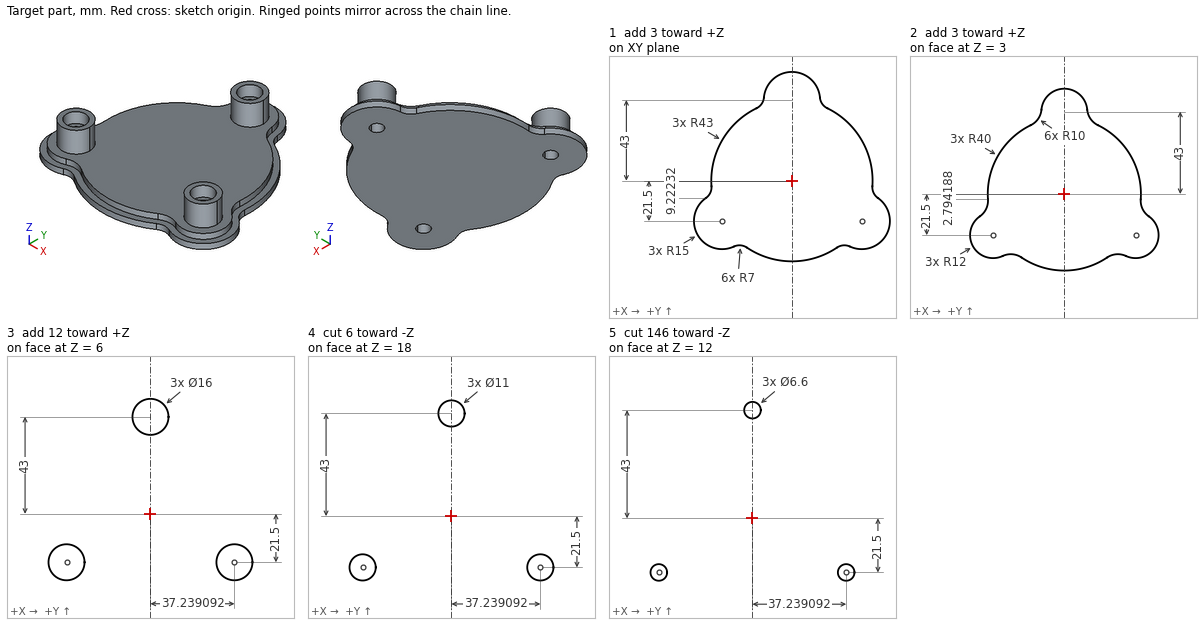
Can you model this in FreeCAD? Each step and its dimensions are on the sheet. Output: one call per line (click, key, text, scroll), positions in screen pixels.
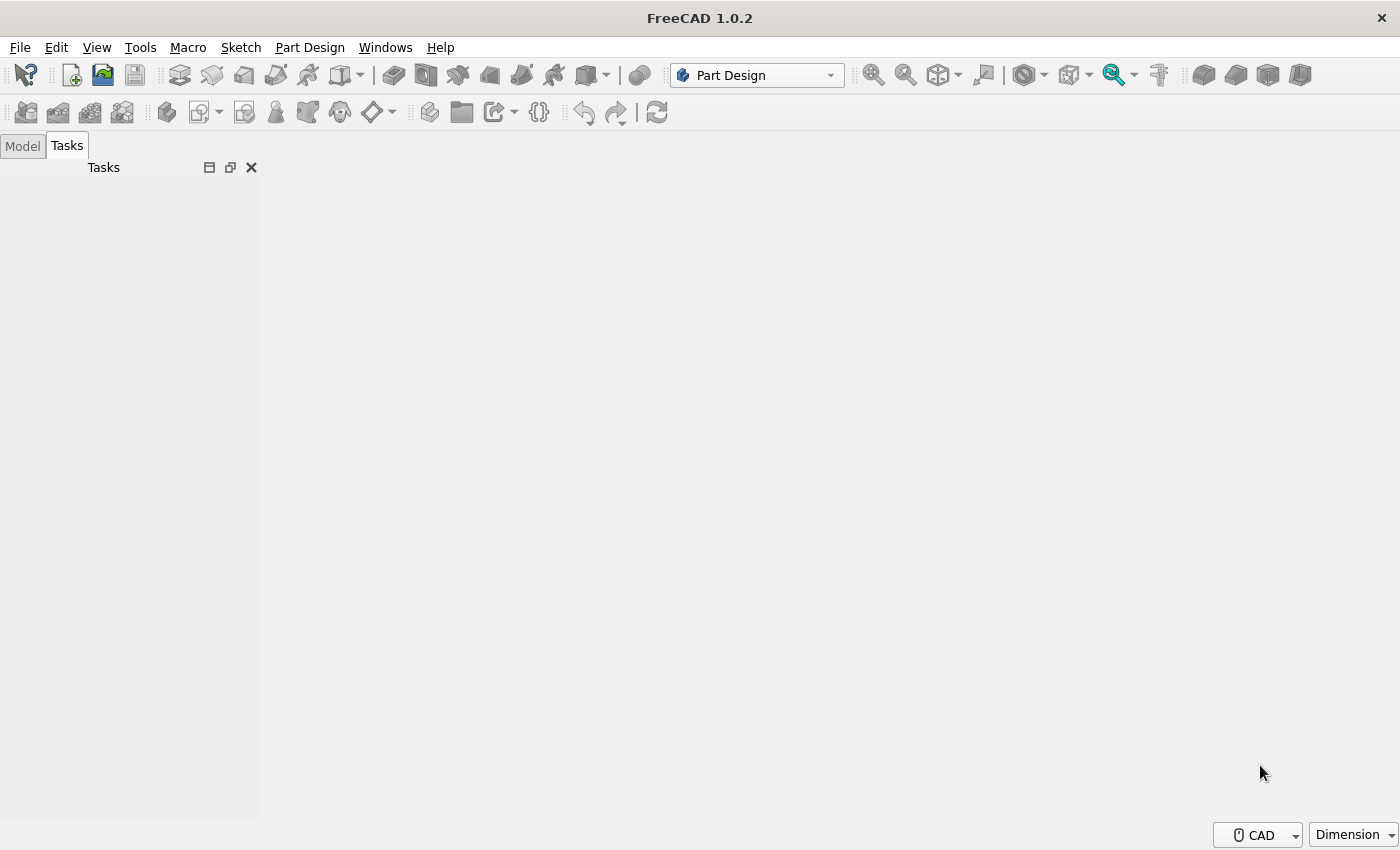
click(72, 76)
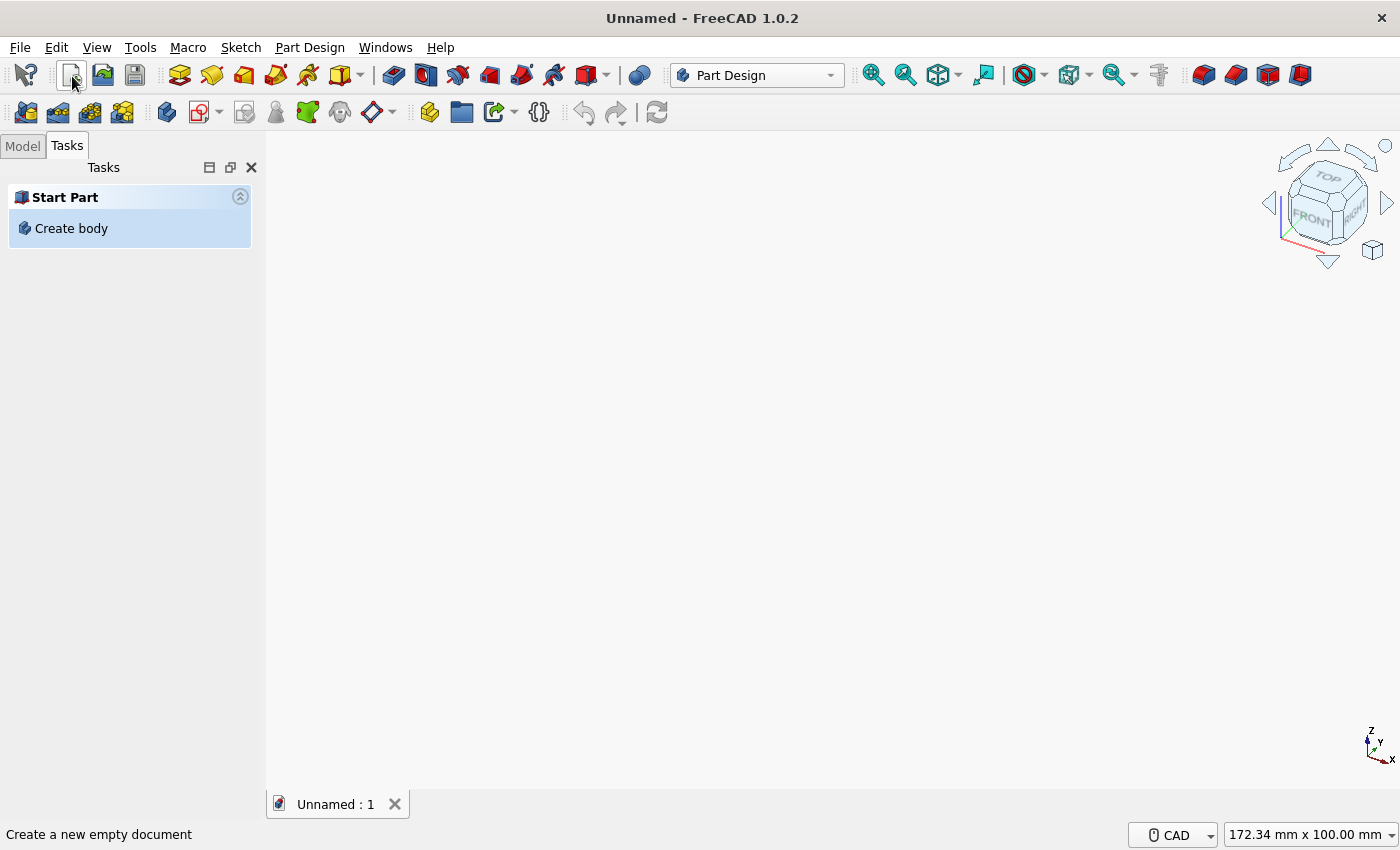
click(200, 112)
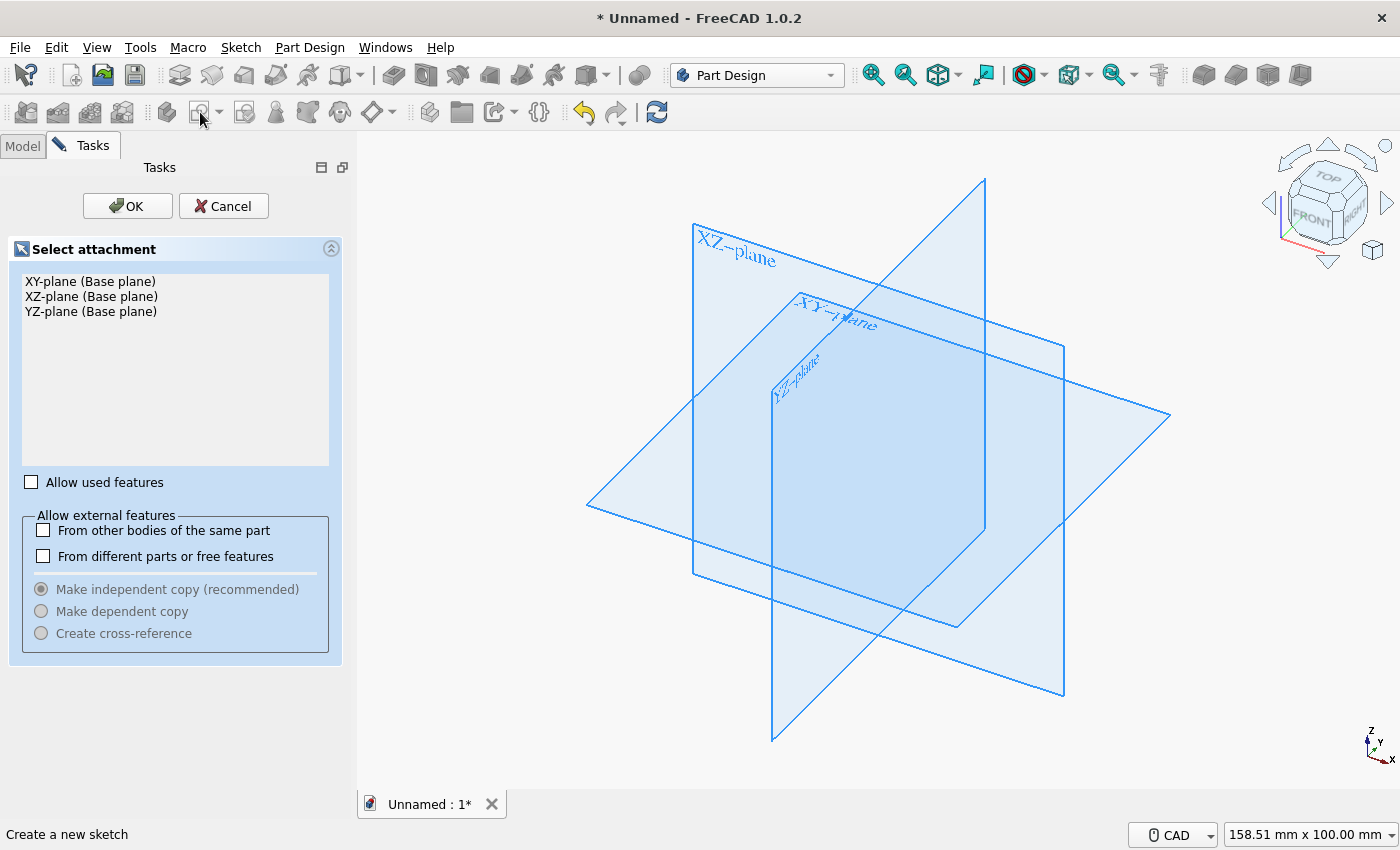
click(82, 282)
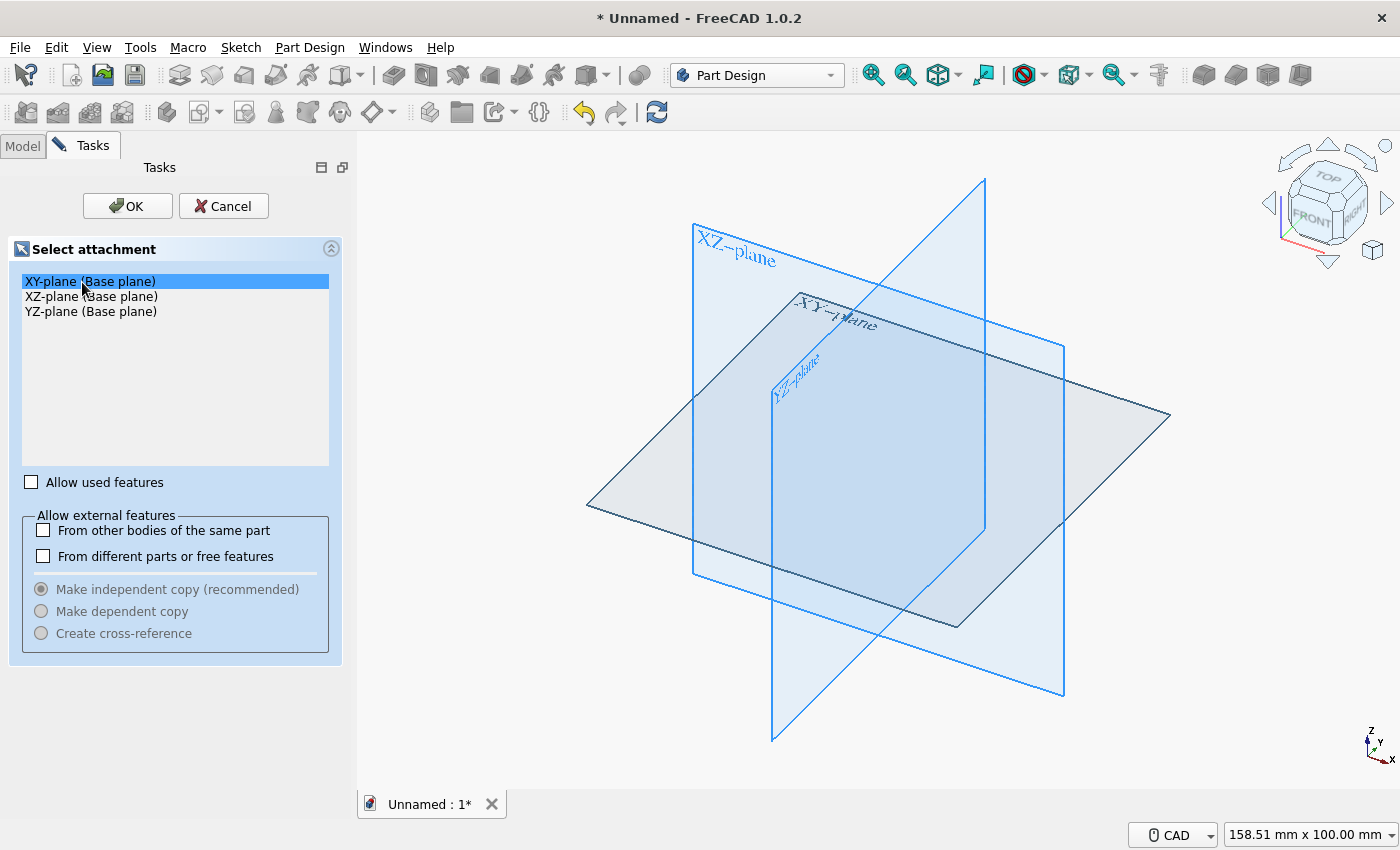
click(128, 206)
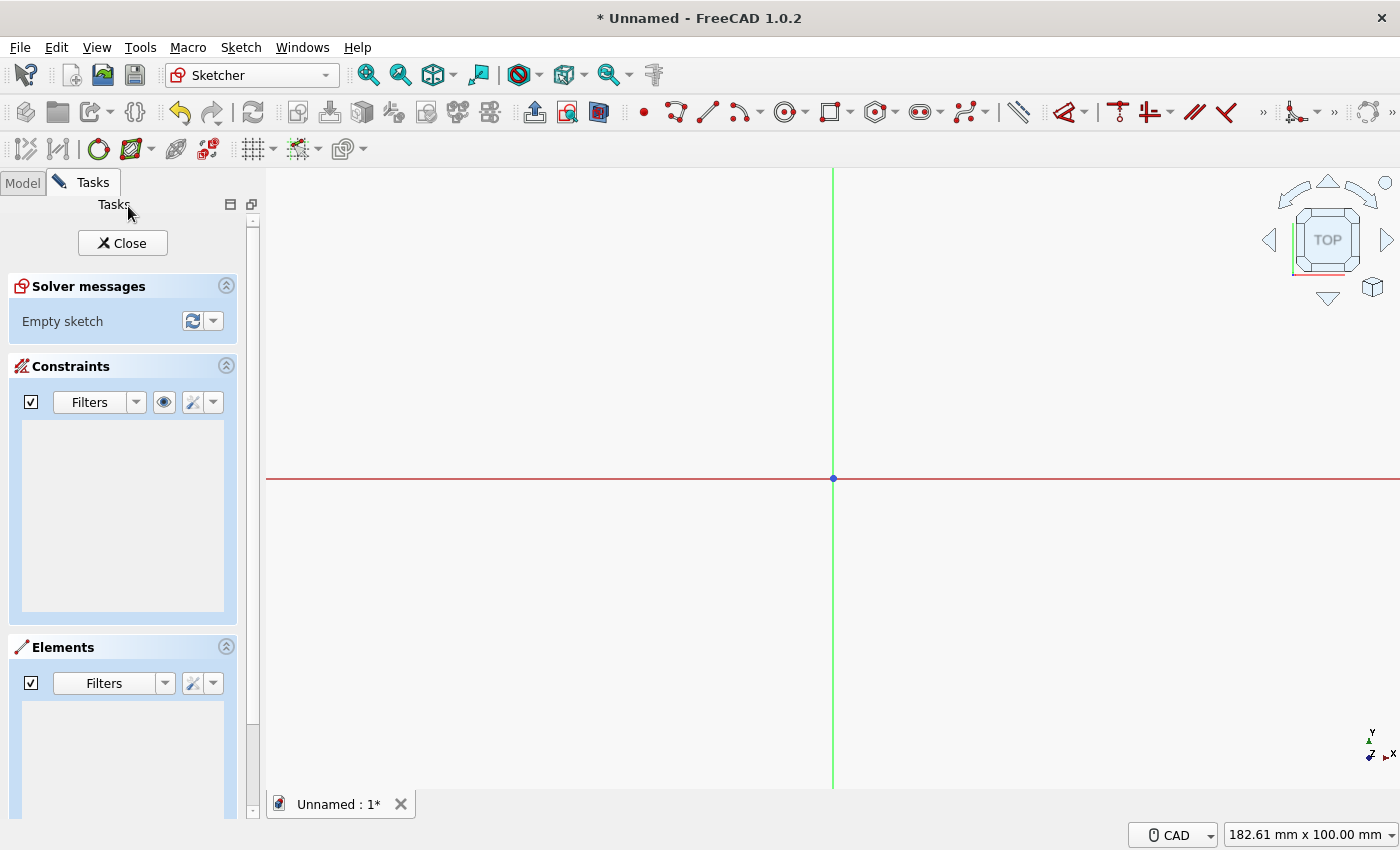
scroll(625, 573, down, 2)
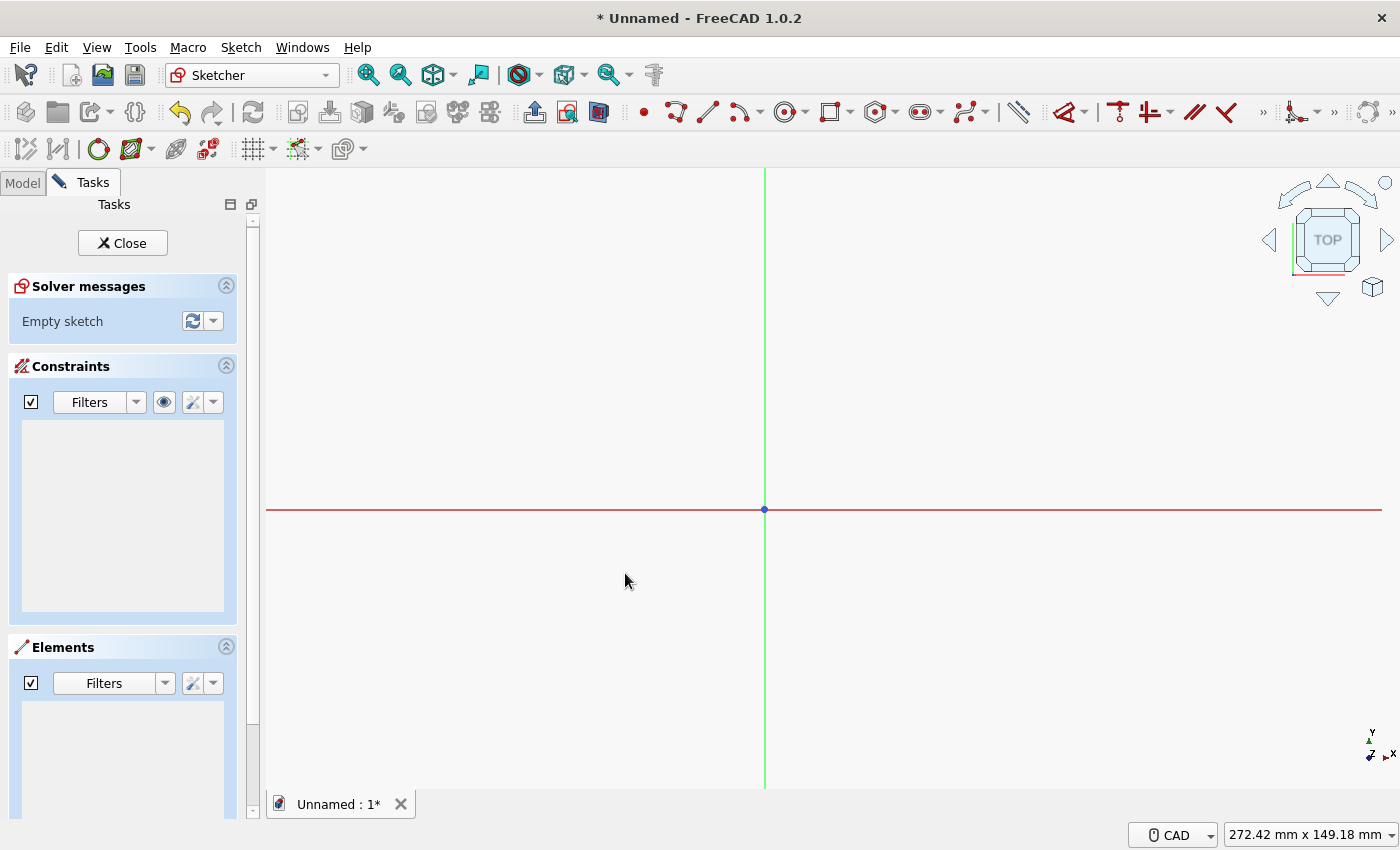
click(762, 112)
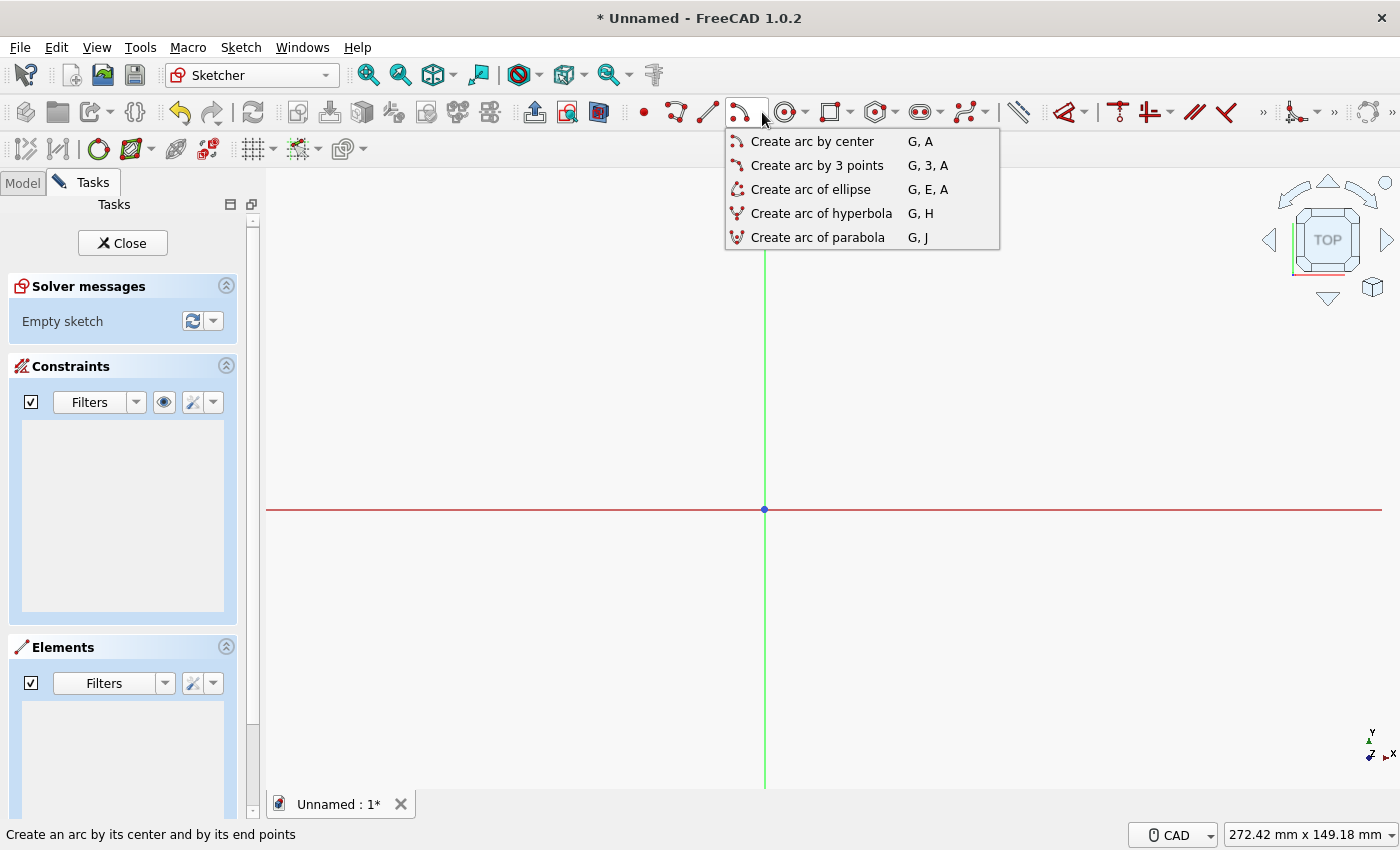
click(862, 165)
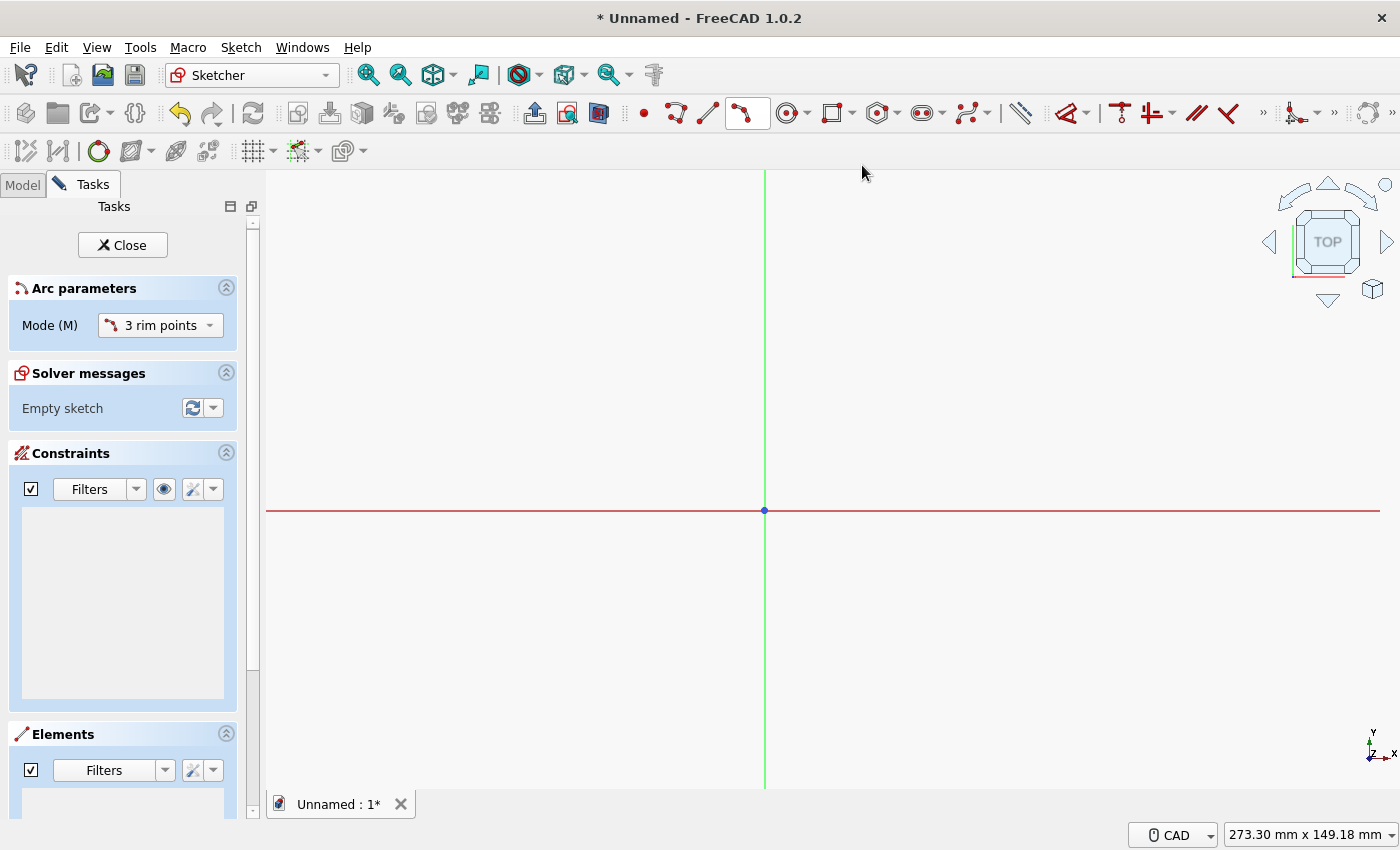
scroll(587, 523, up, 2)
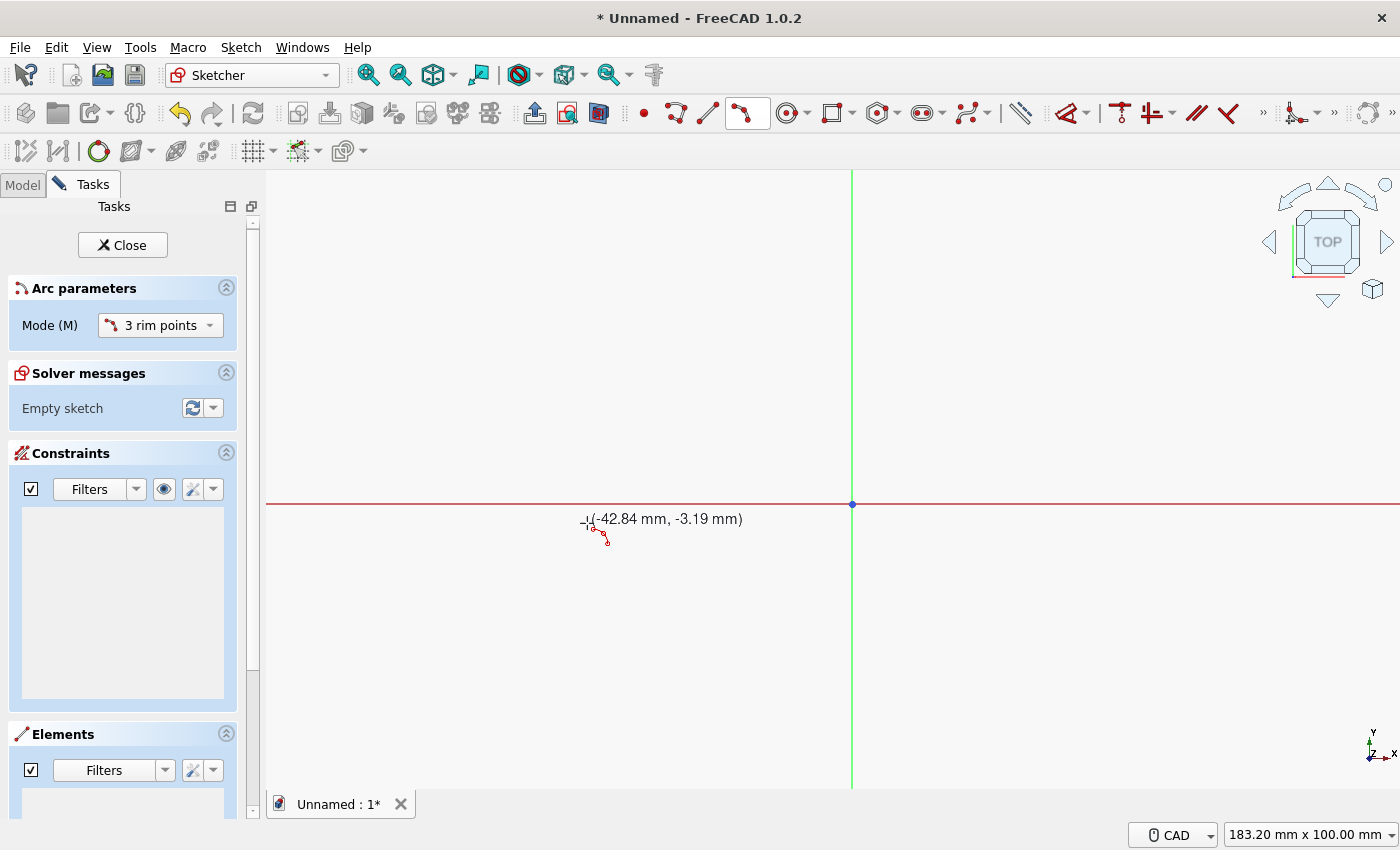
click(587, 523)
click(568, 562)